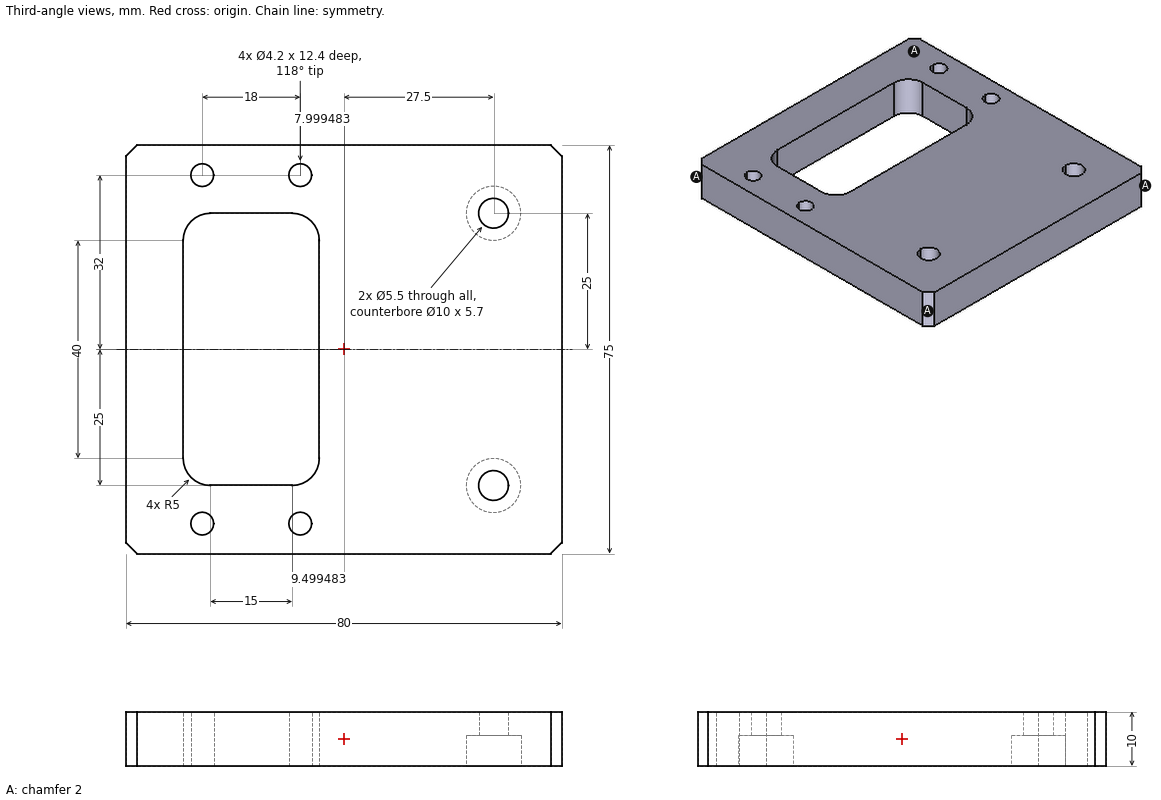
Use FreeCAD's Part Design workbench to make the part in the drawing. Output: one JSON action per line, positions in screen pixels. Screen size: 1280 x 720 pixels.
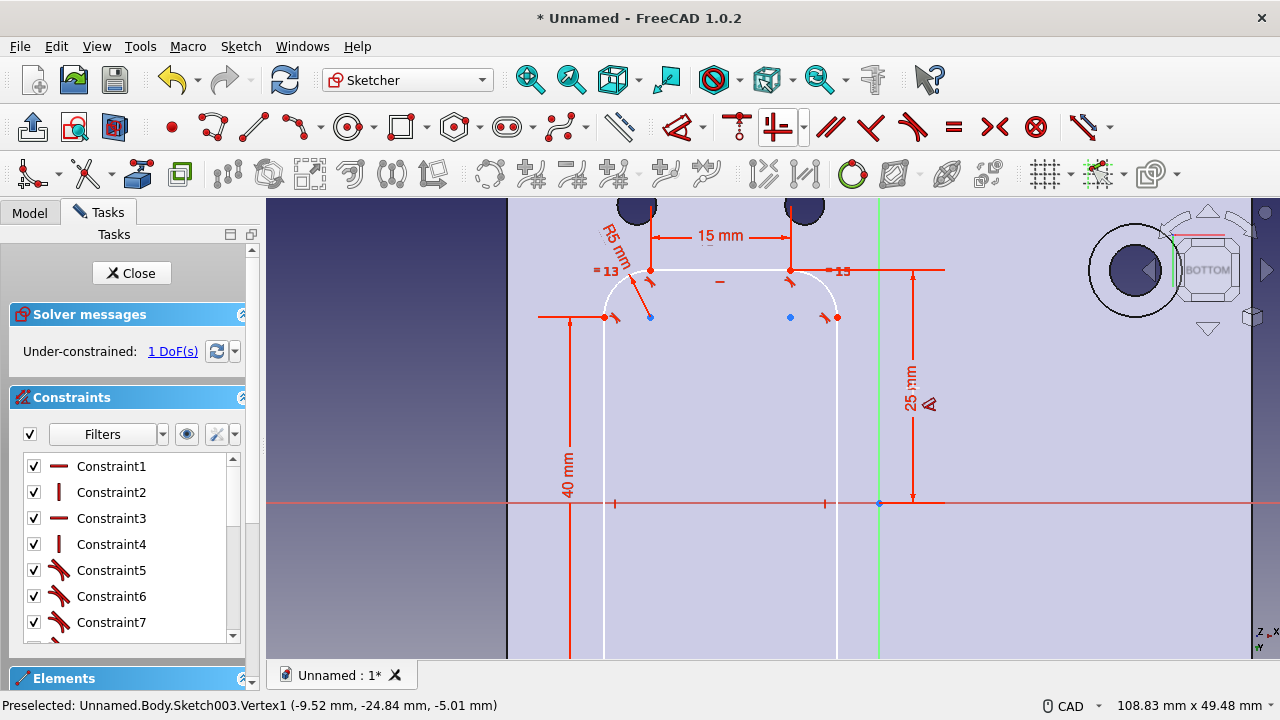
{"action": "left_click", "coordinate": [791, 270]}
{"action": "left_click", "coordinate": [835, 236]}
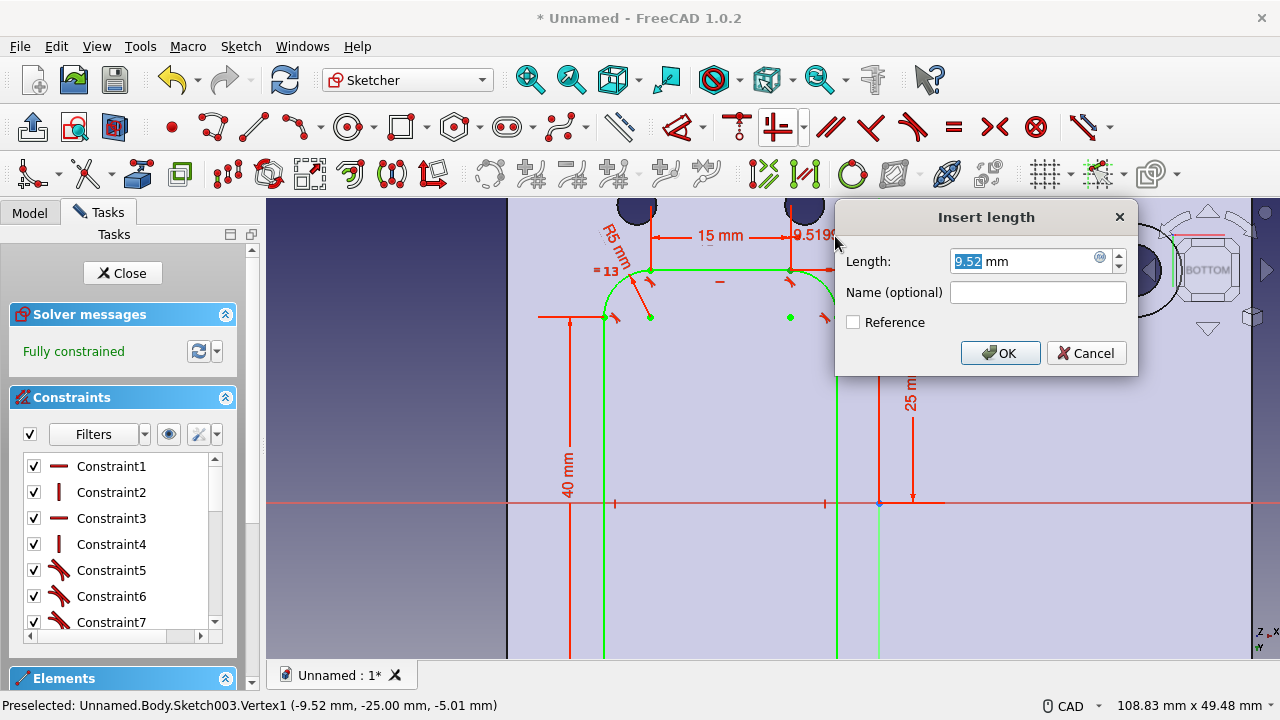
{"action": "type", "text": "9.499483"}
{"action": "key", "text": "Return"}
{"action": "key", "text": "Escape"}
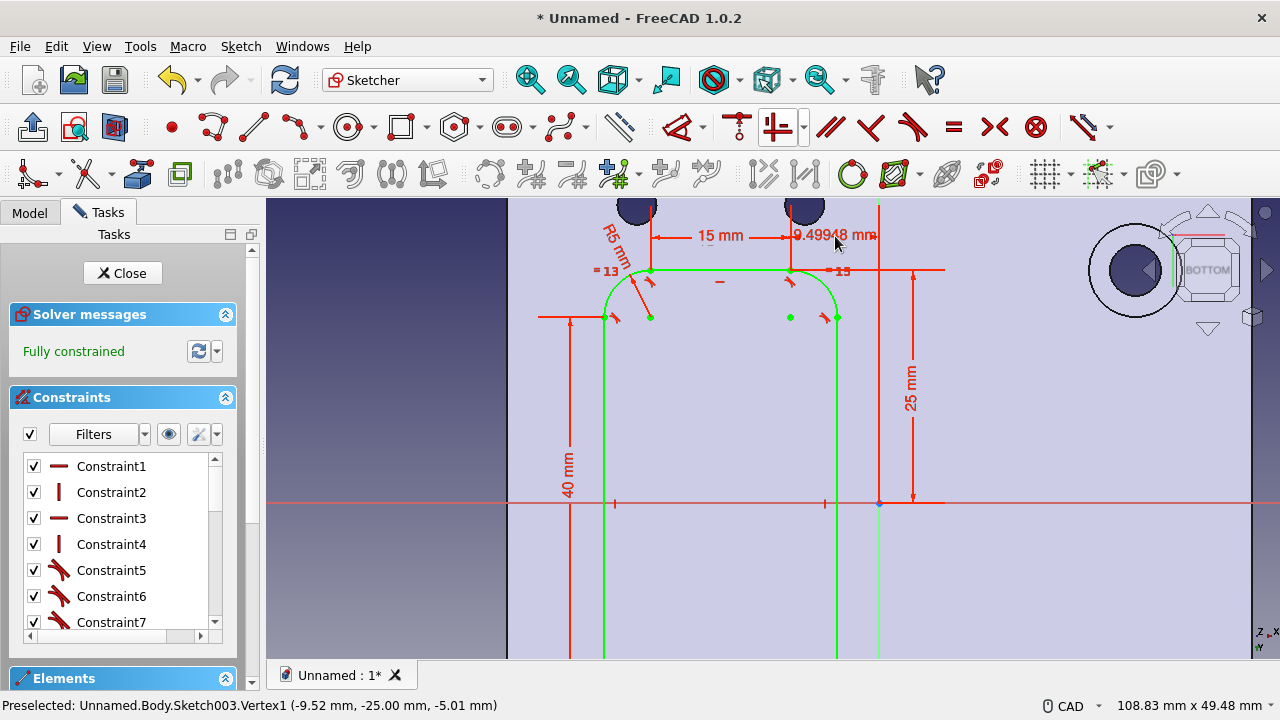
{"action": "left_click", "coordinate": [123, 273]}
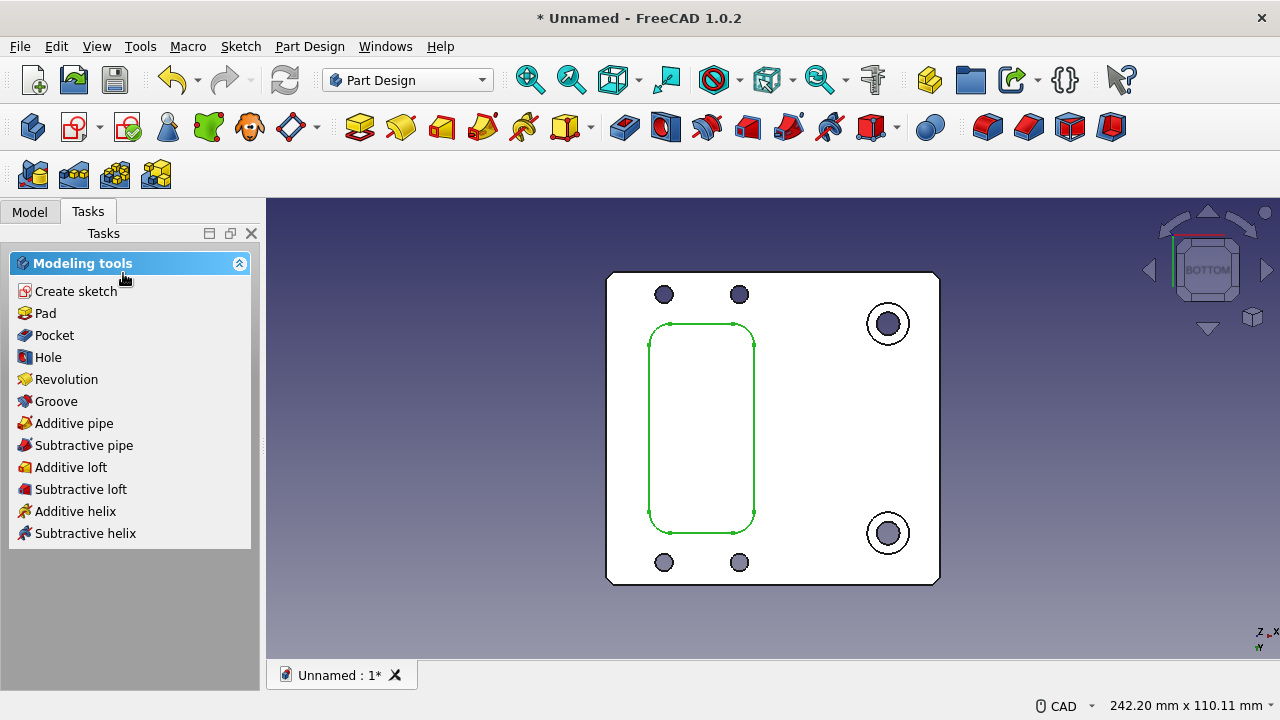
{"action": "left_click", "coordinate": [625, 128]}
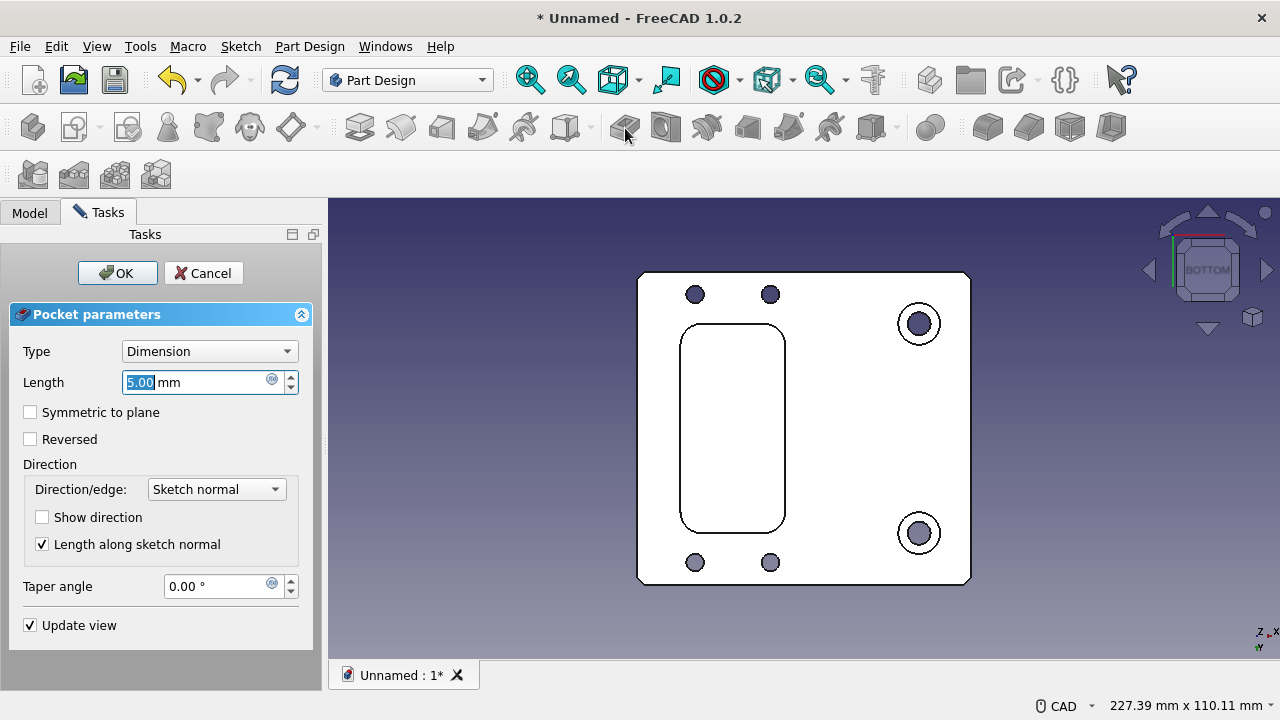
{"action": "left_click", "coordinate": [210, 352]}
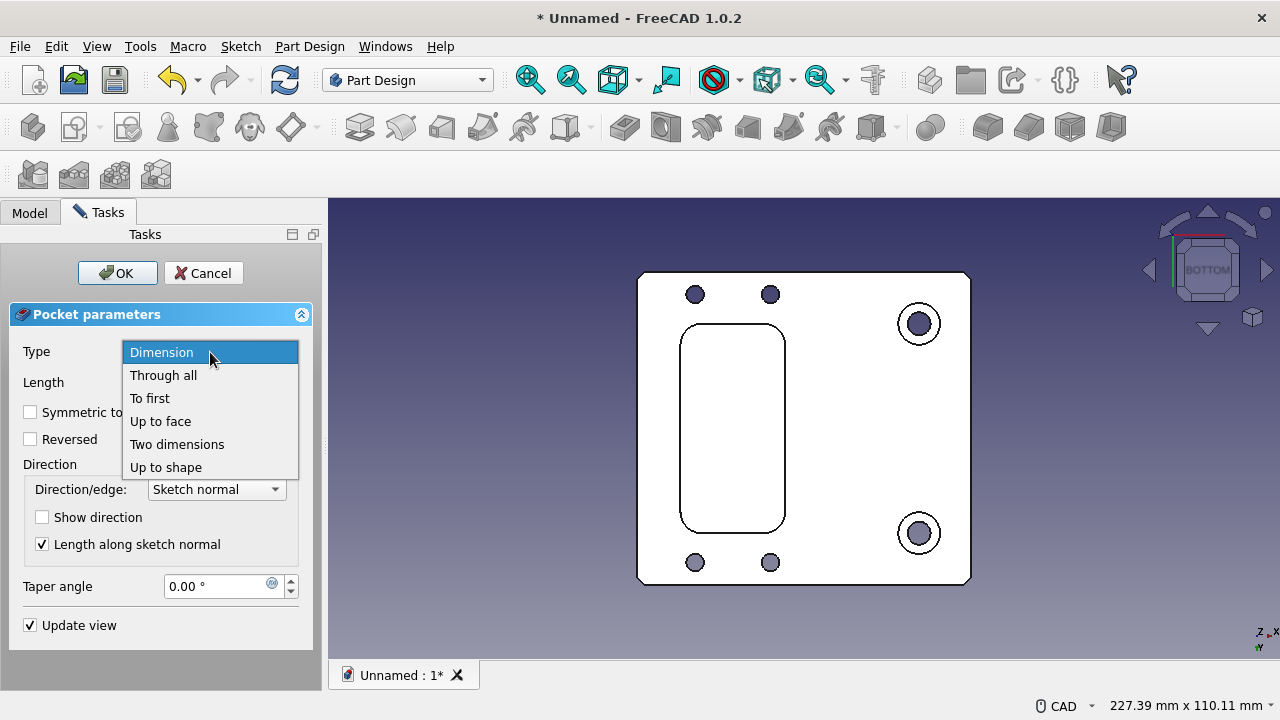
{"action": "left_click", "coordinate": [208, 376]}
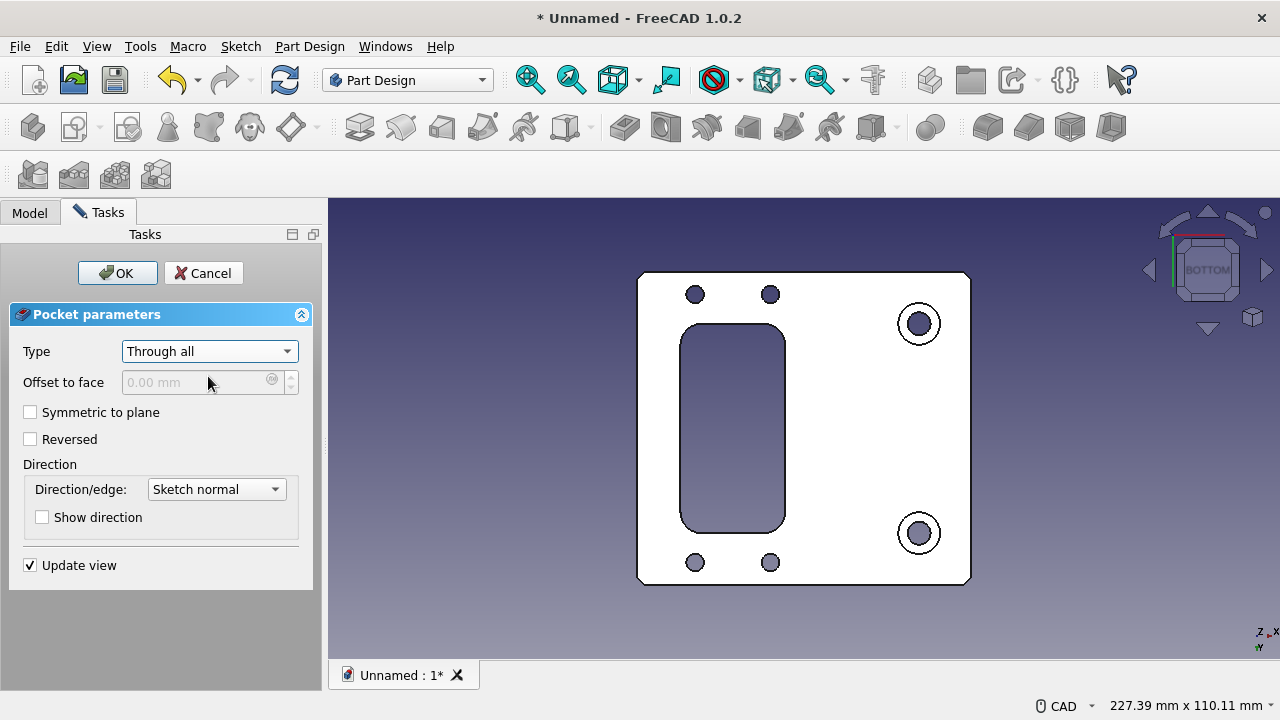
{"action": "left_click", "coordinate": [118, 273]}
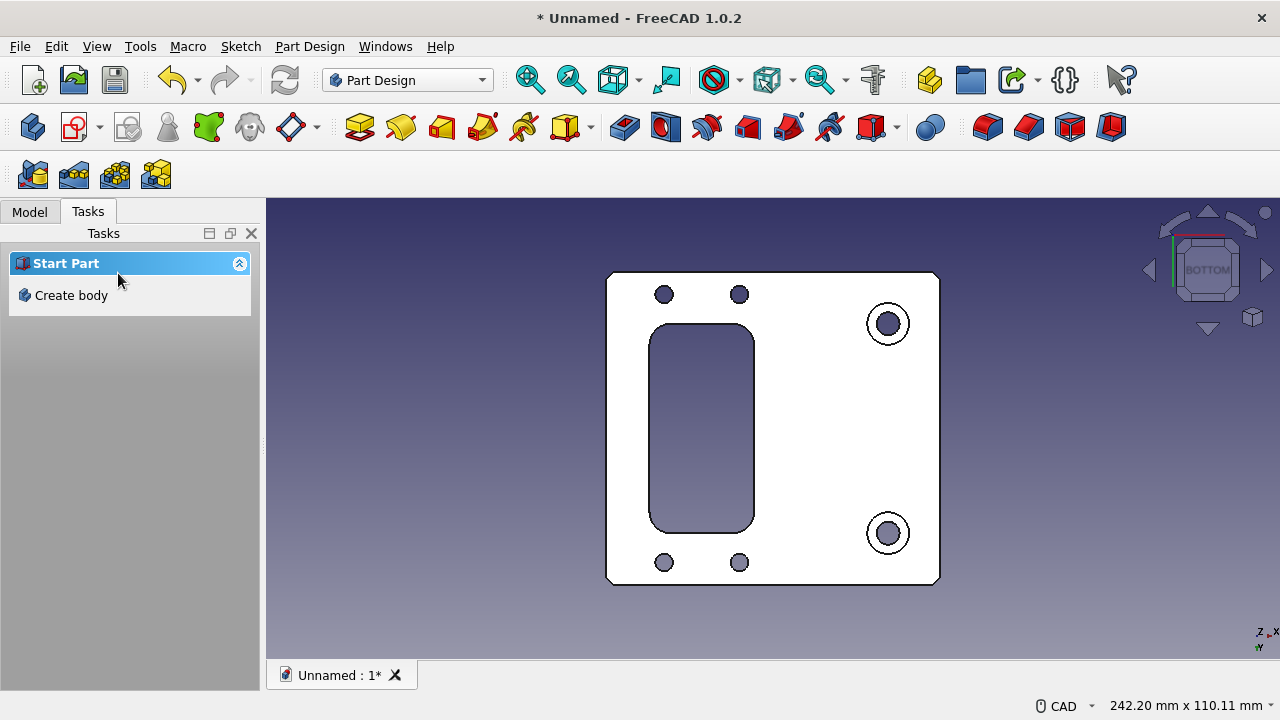
{"action": "key", "text": "0"}